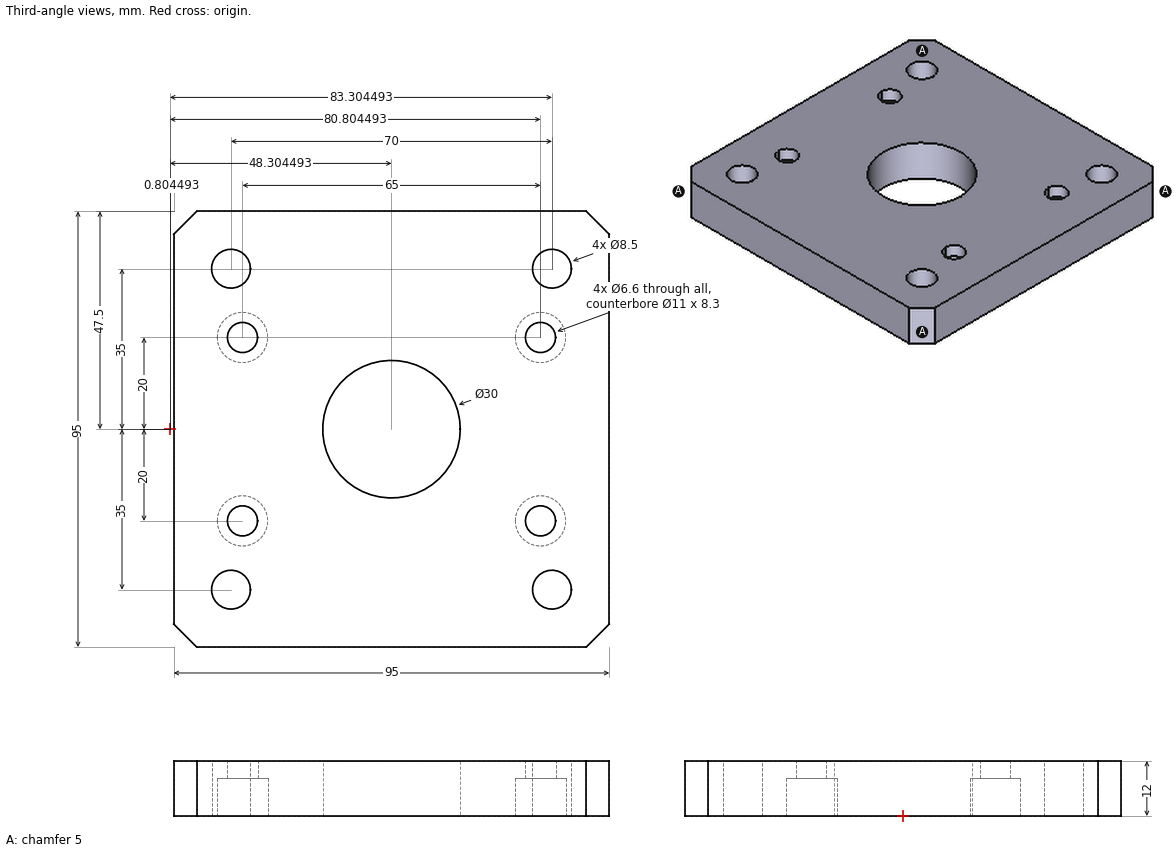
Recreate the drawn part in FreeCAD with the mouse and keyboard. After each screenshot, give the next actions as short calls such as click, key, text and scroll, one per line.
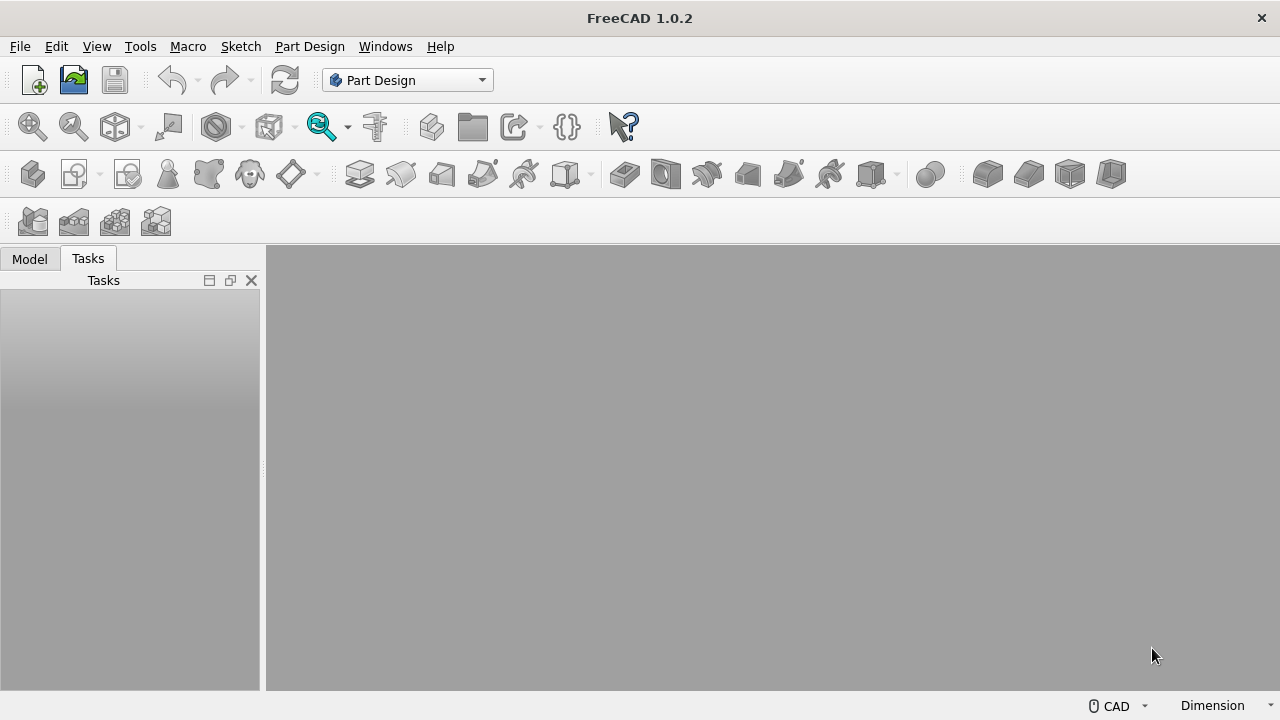
key(ctrl+n)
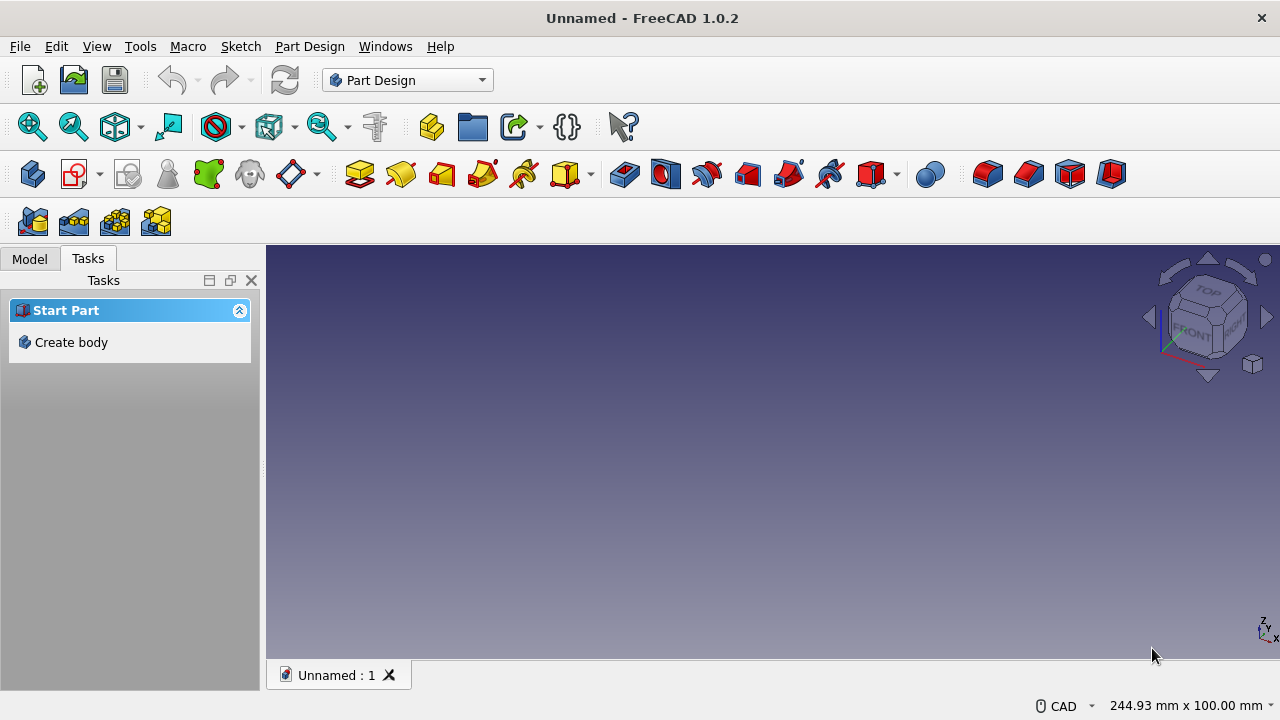
click(74, 174)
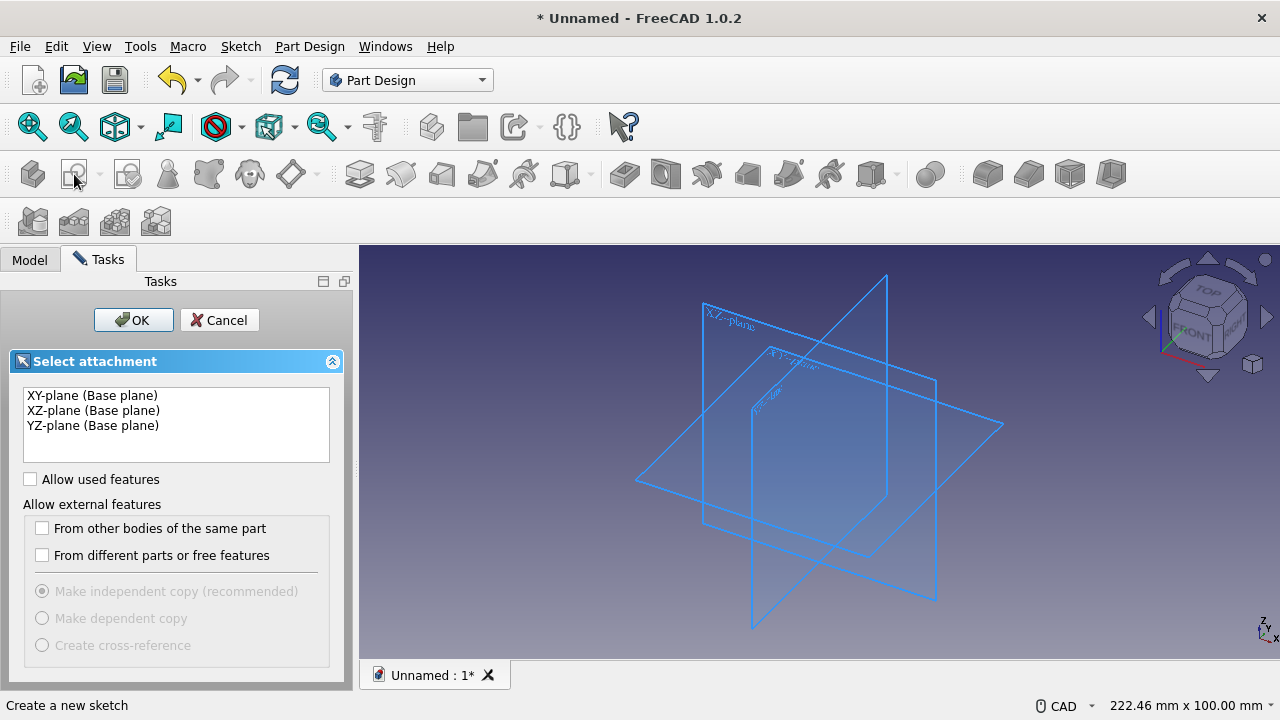
click(84, 396)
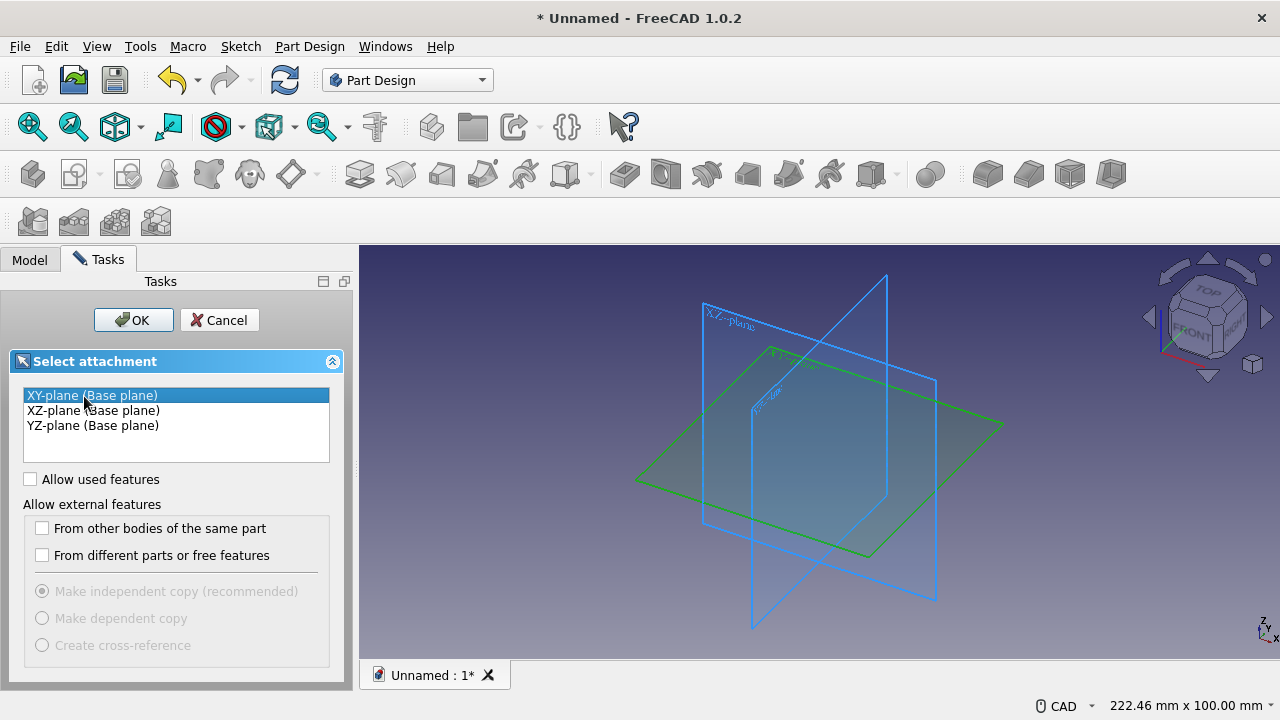
click(134, 320)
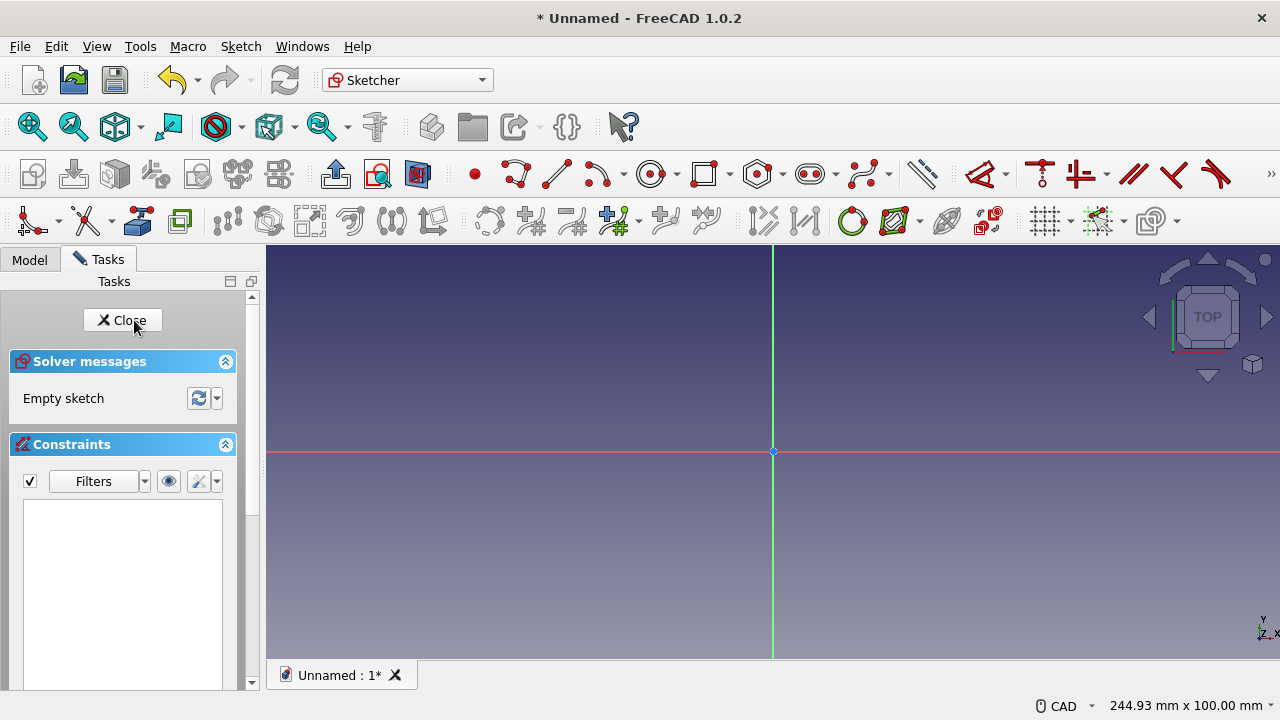
scroll(294, 452, down, 2)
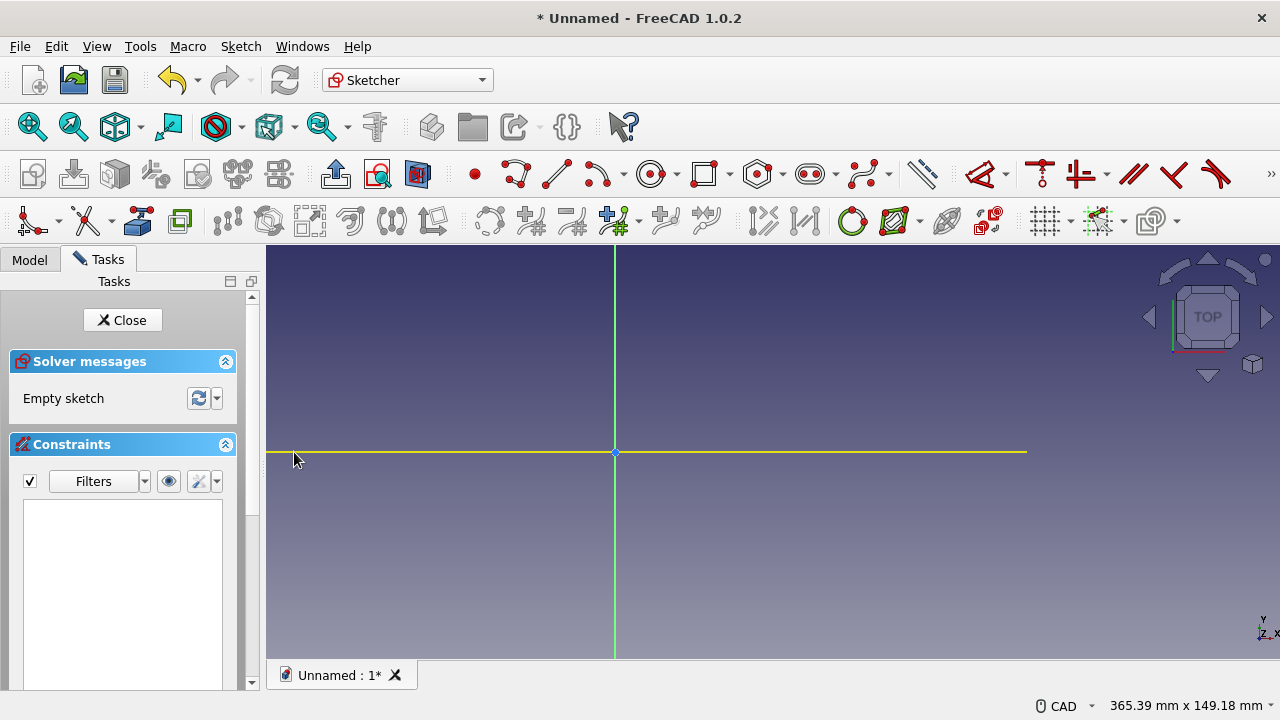
key(g)
key(r)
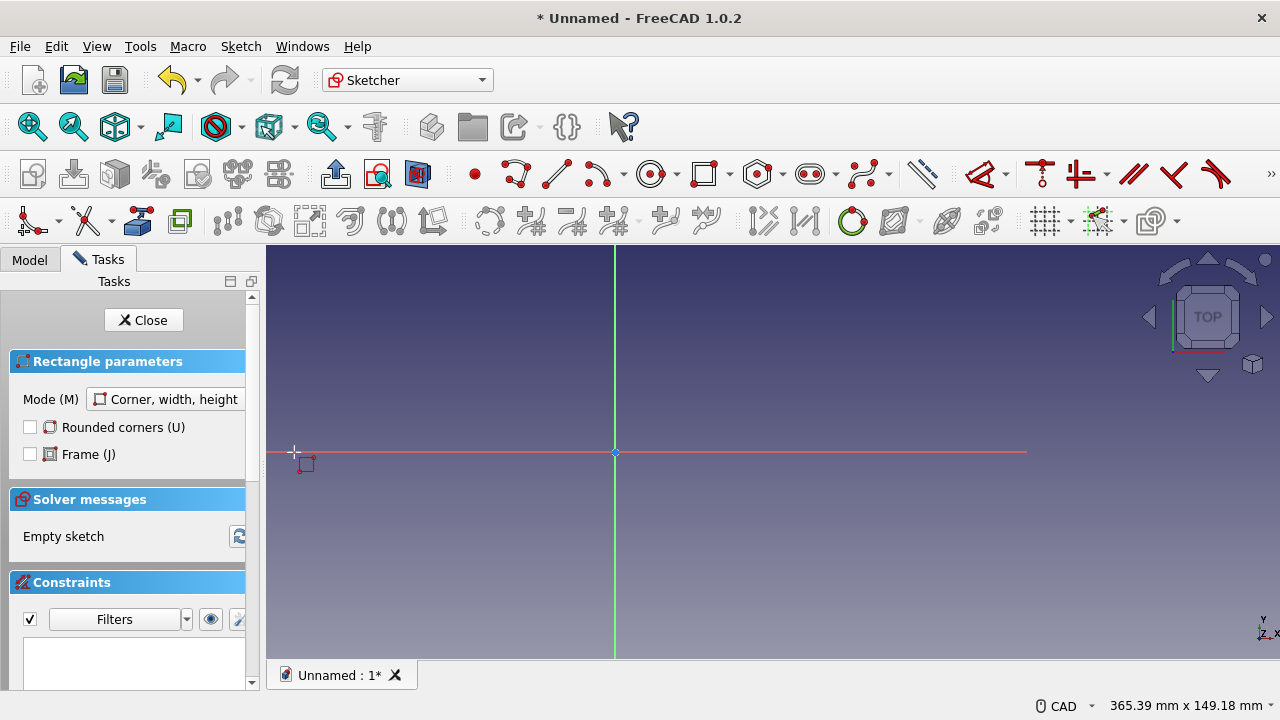
scroll(617, 320, up, 10)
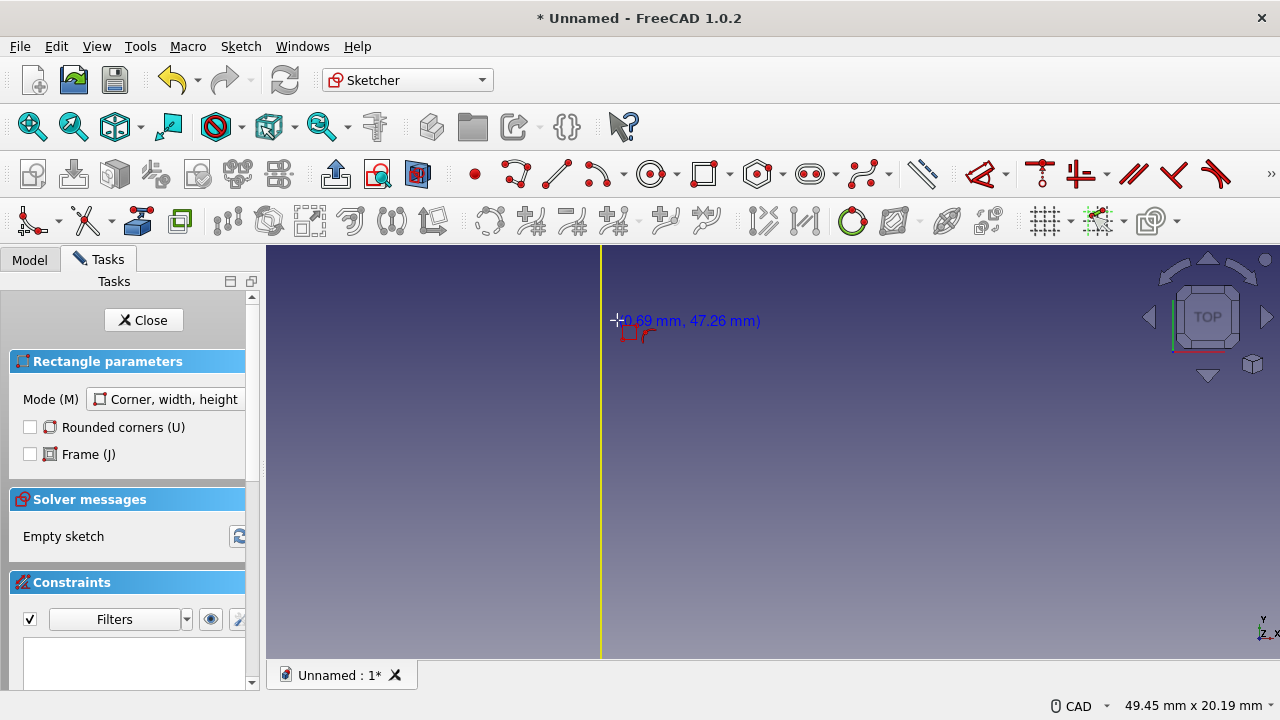
click(617, 321)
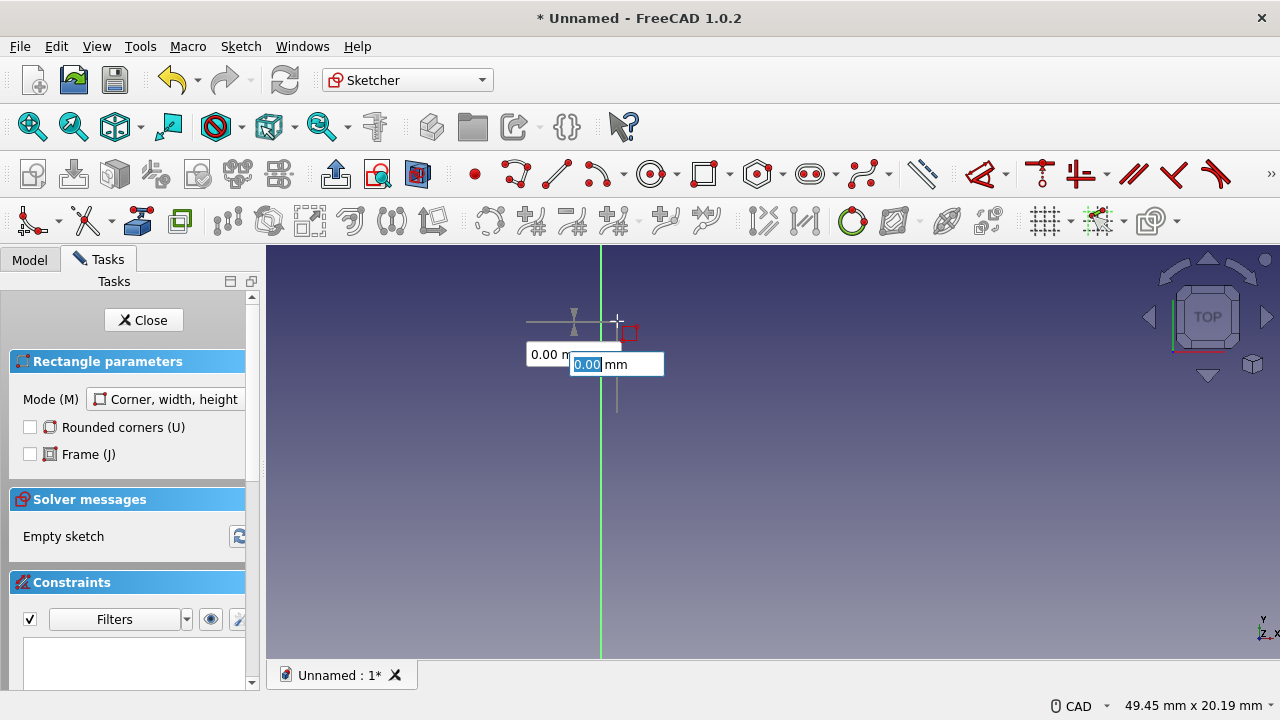
scroll(567, 320, down, 10)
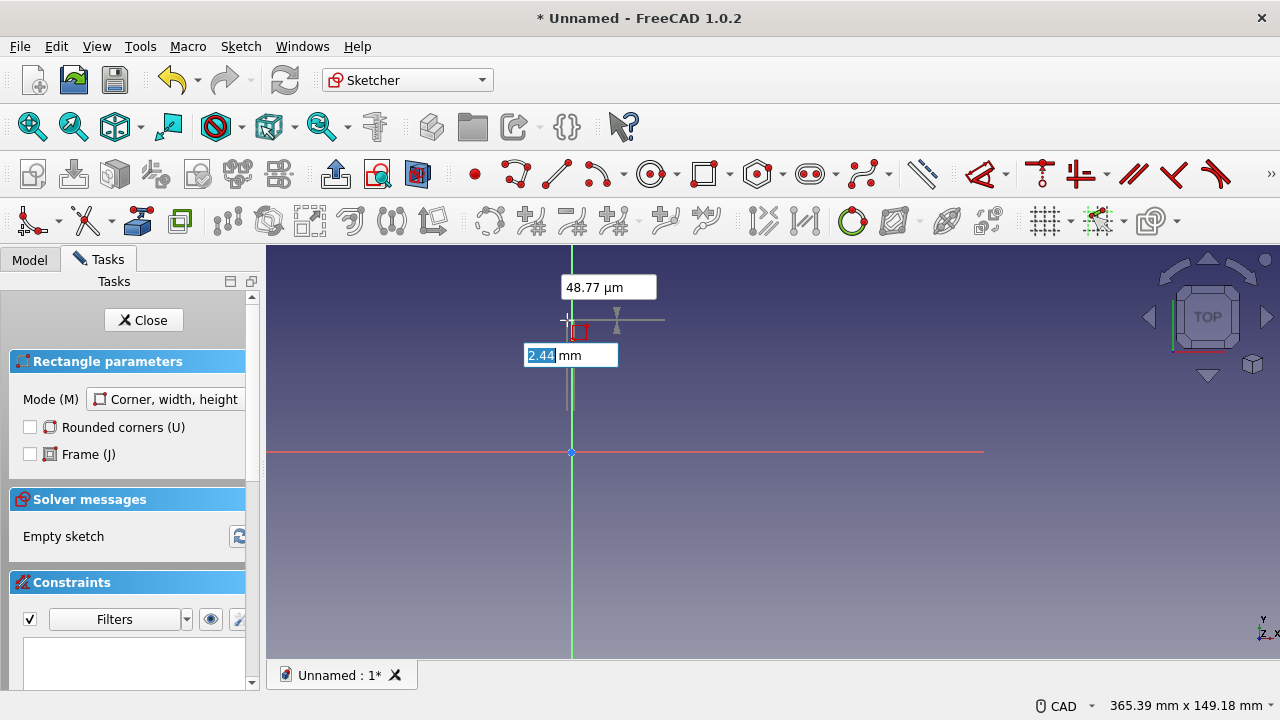
click(838, 584)
key(Escape)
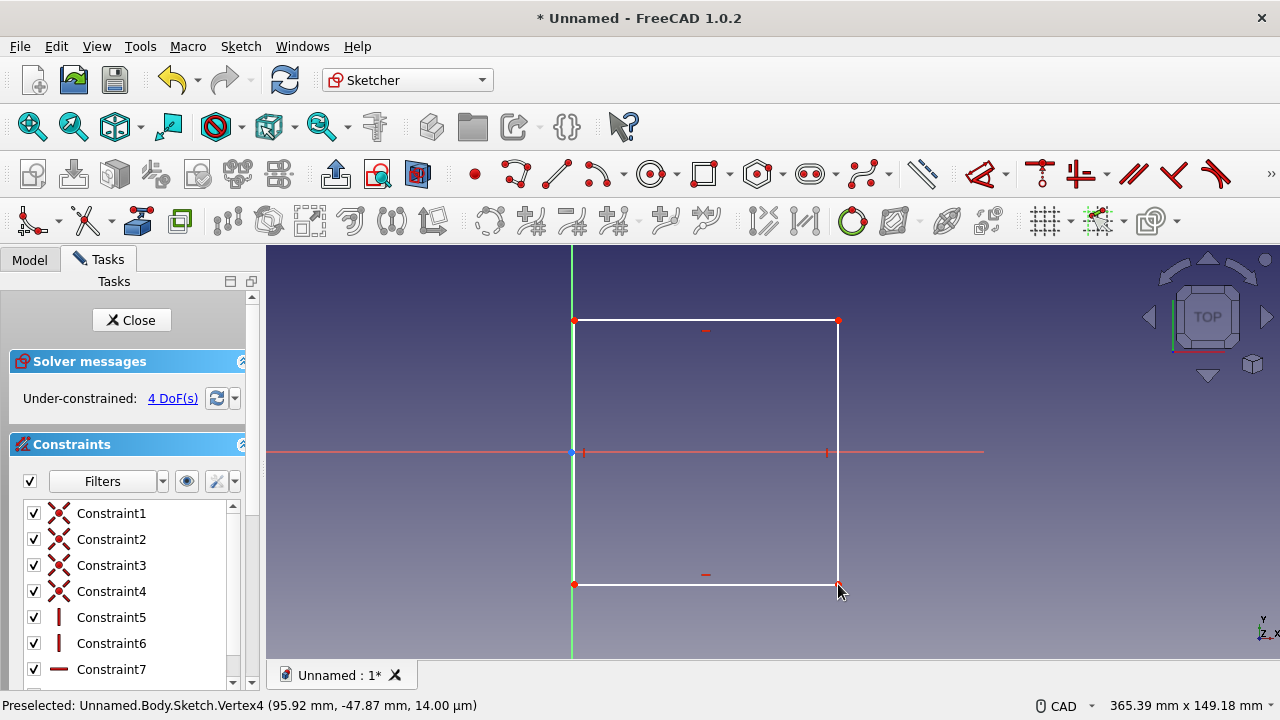
key(d)